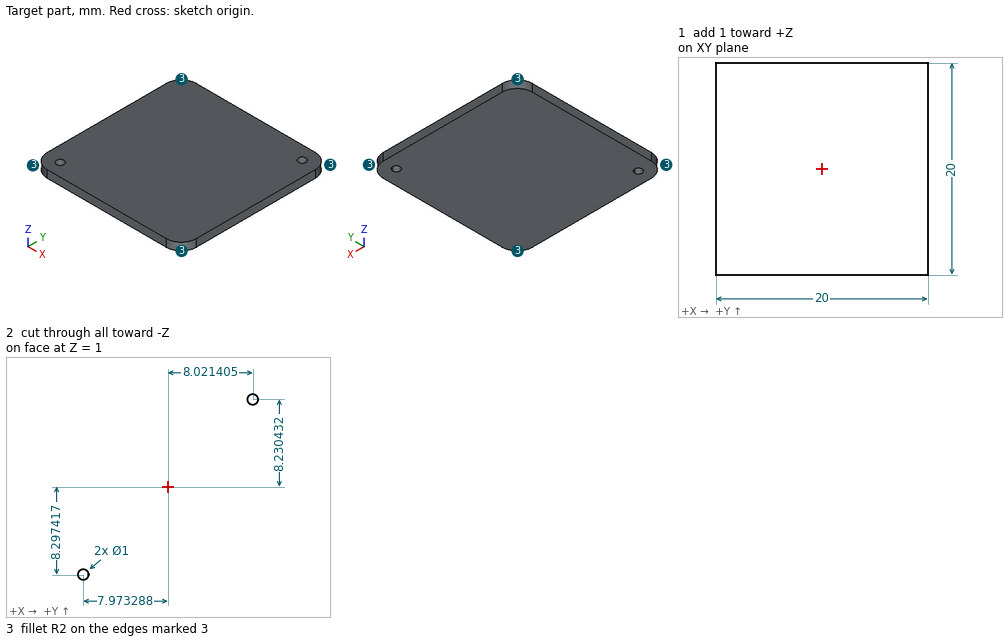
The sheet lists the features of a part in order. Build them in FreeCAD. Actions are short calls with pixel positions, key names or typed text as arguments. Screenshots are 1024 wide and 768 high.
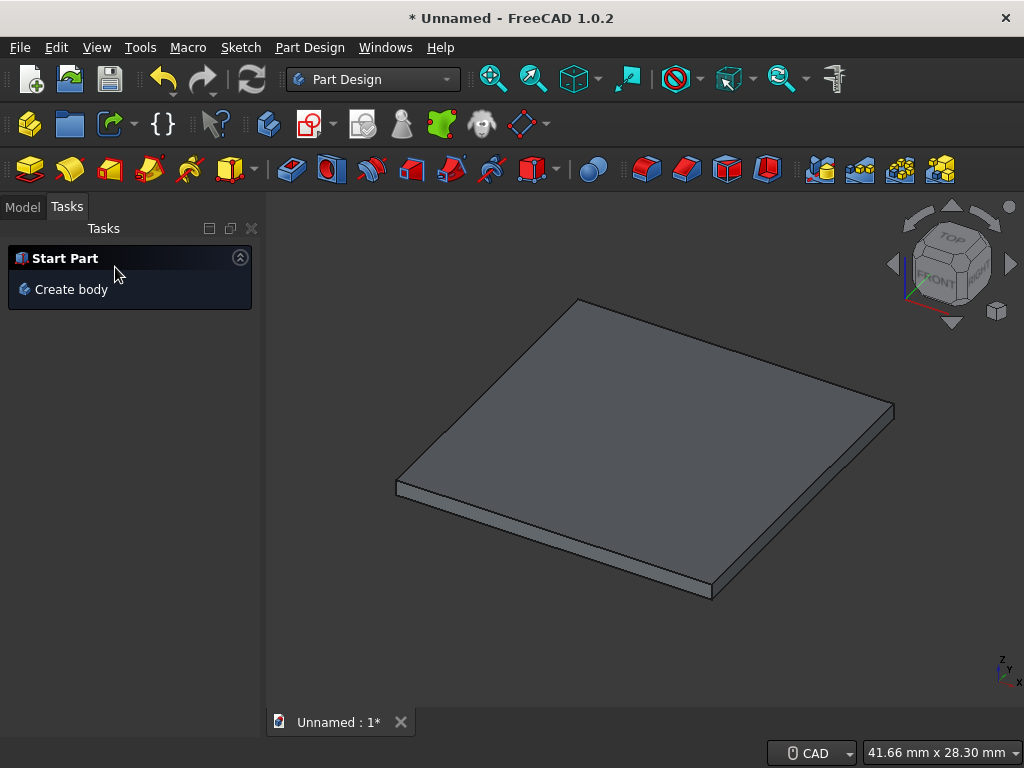
click(645, 441)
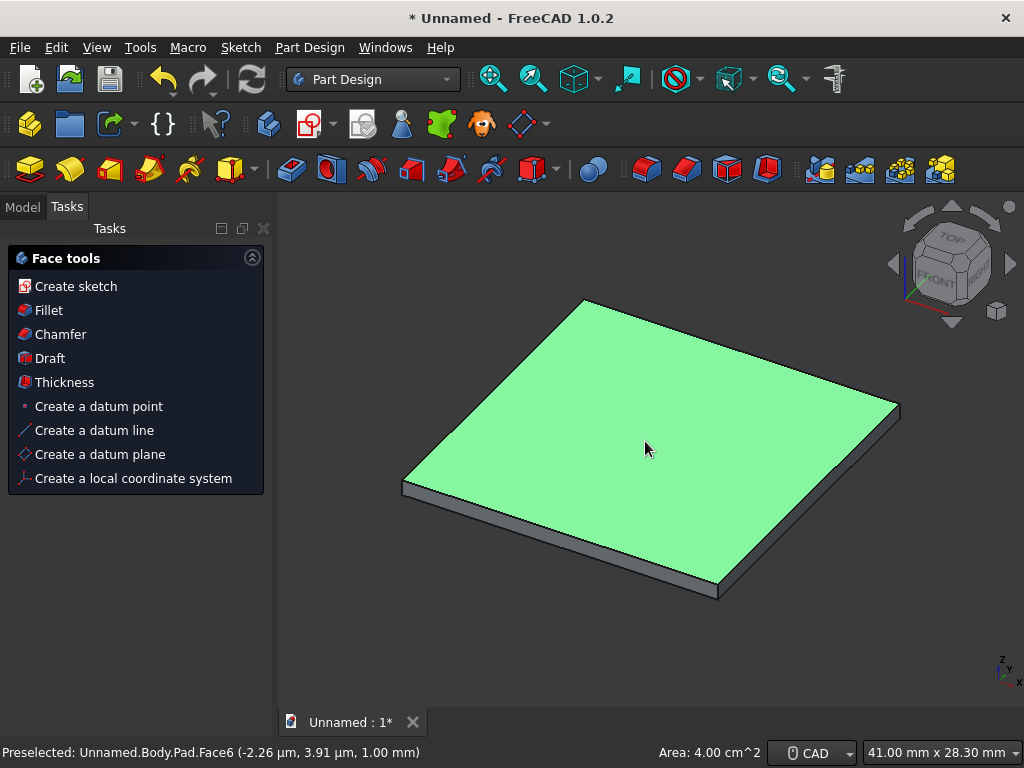
click(310, 124)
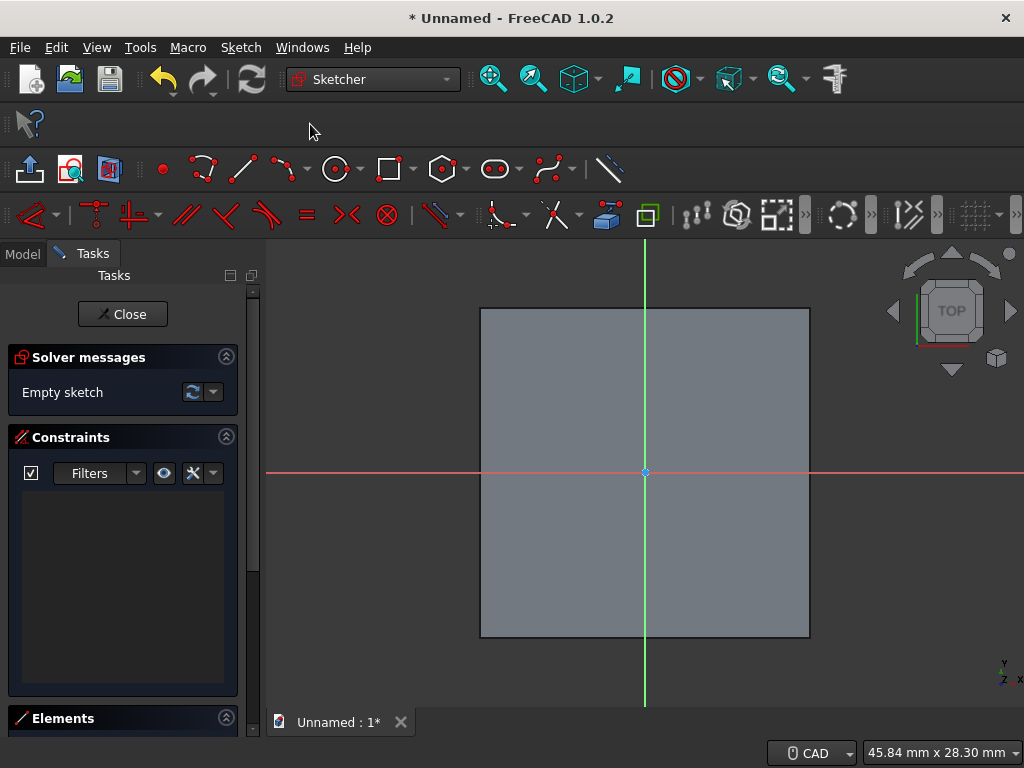
click(336, 170)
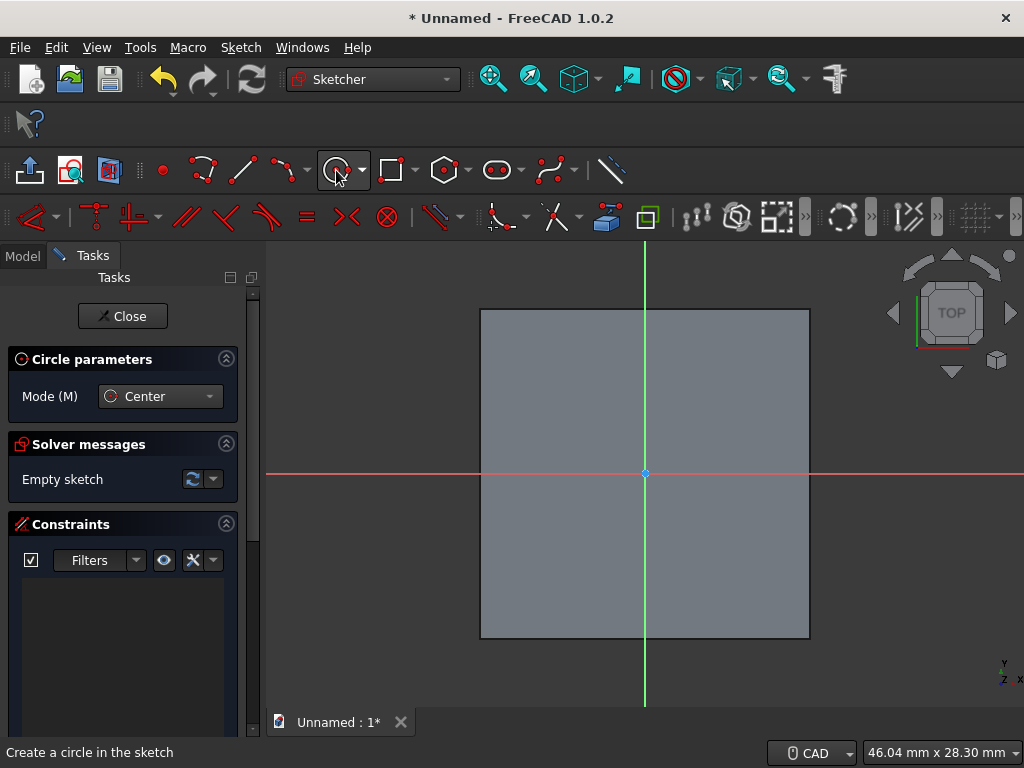
scroll(514, 611, up, 6)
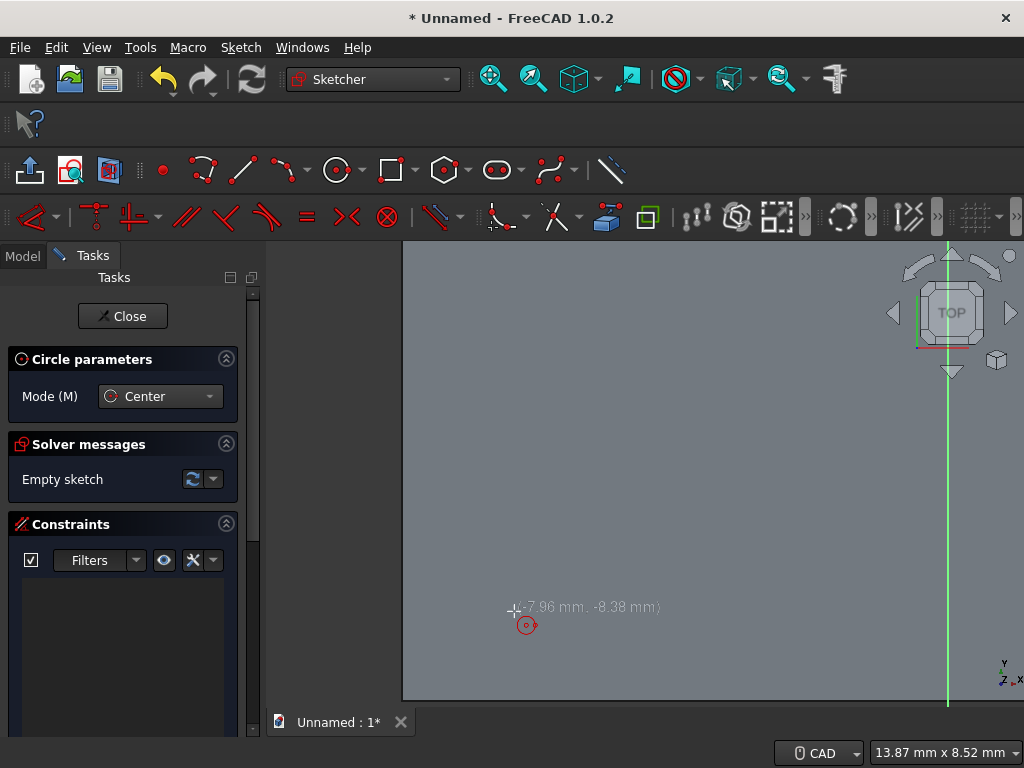
click(512, 608)
move(532, 589)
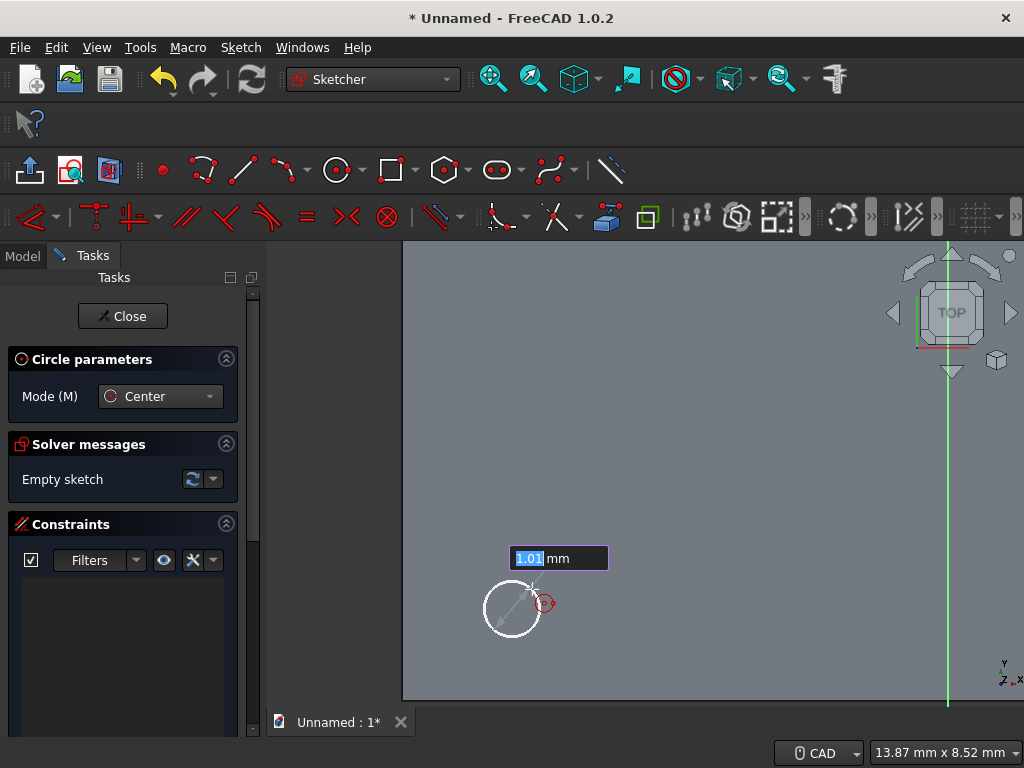
text(1)
key(Return)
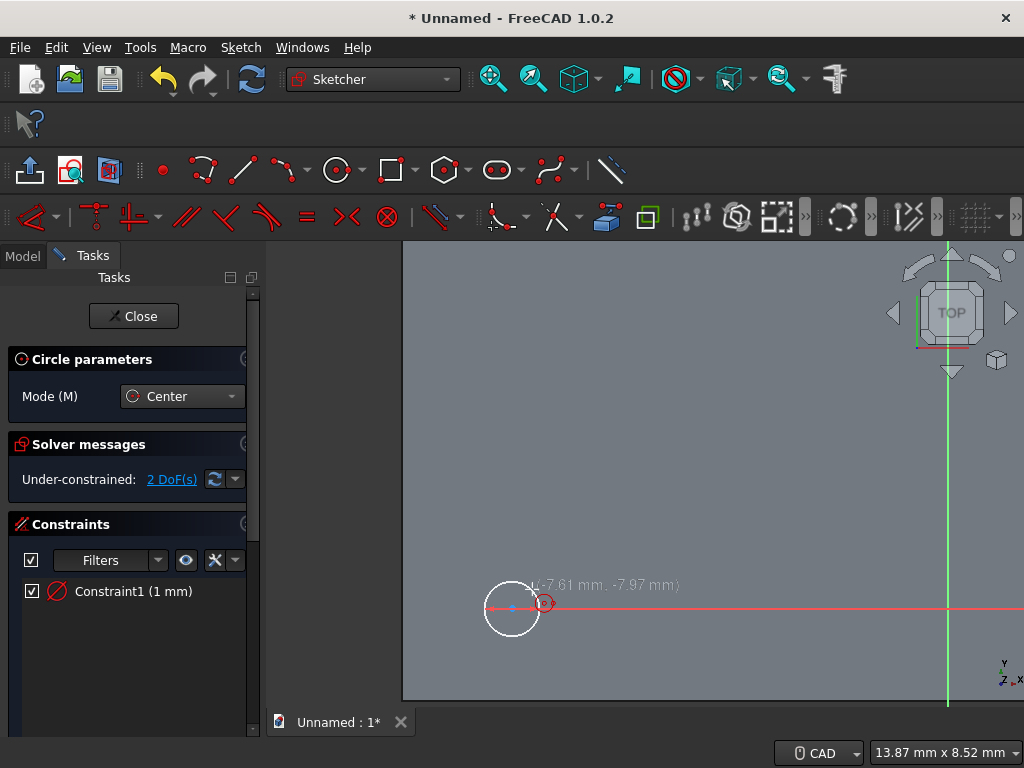
scroll(416, 611, down, 6)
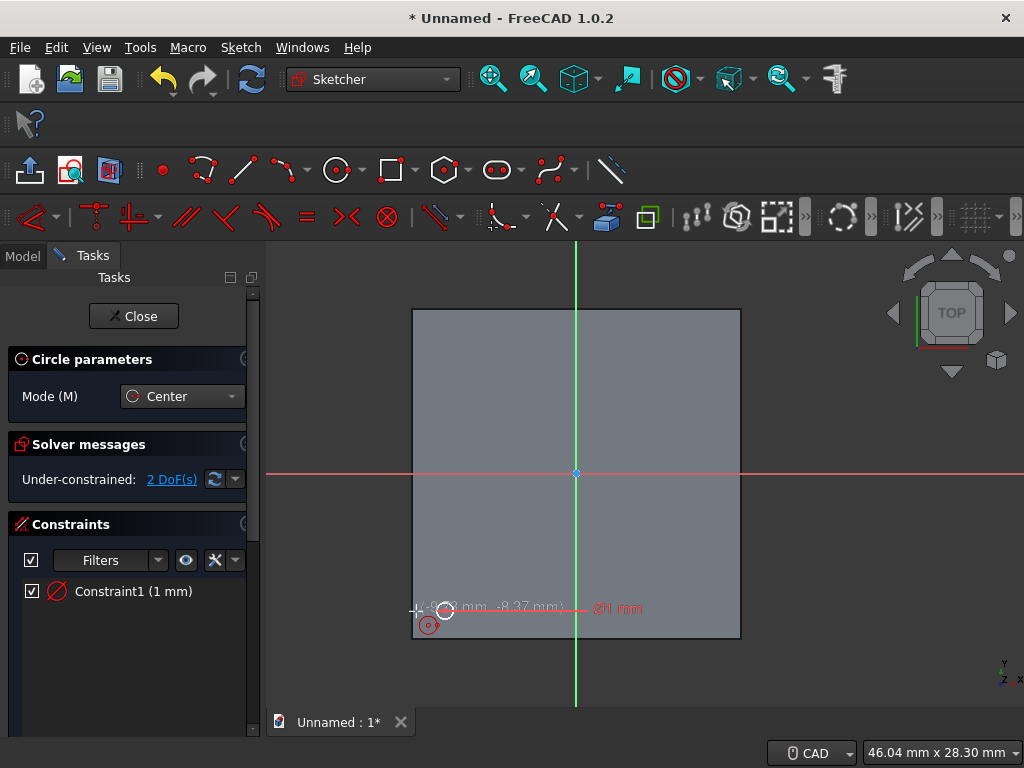
scroll(709, 338, up, 6)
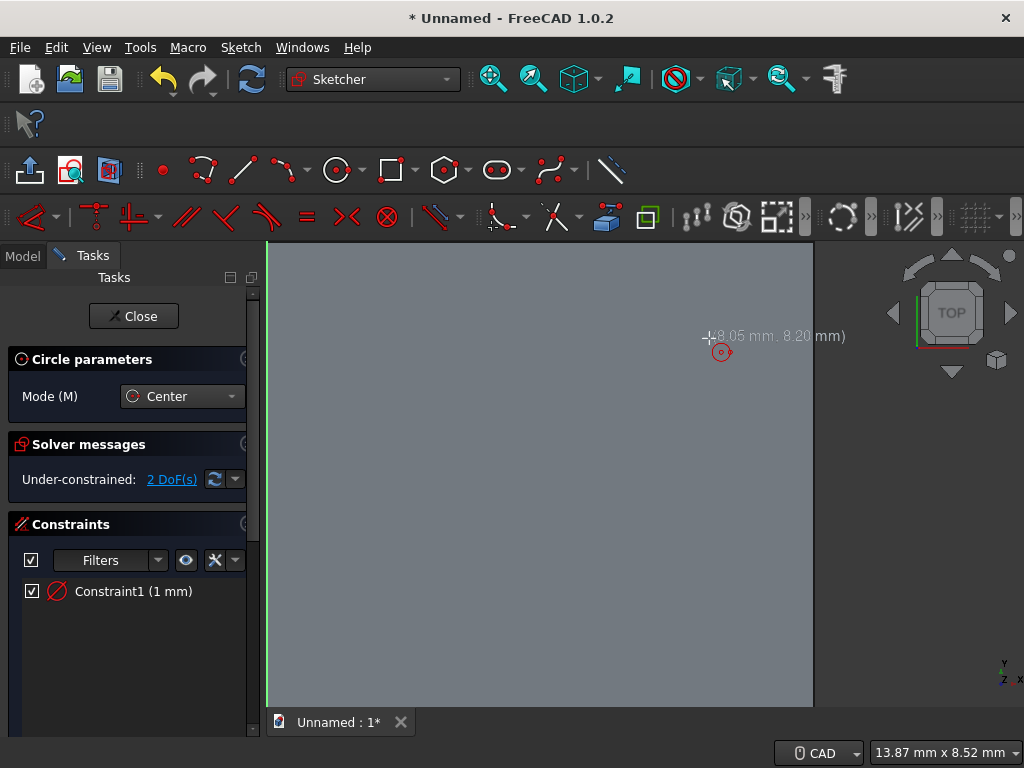
click(706, 339)
move(725, 320)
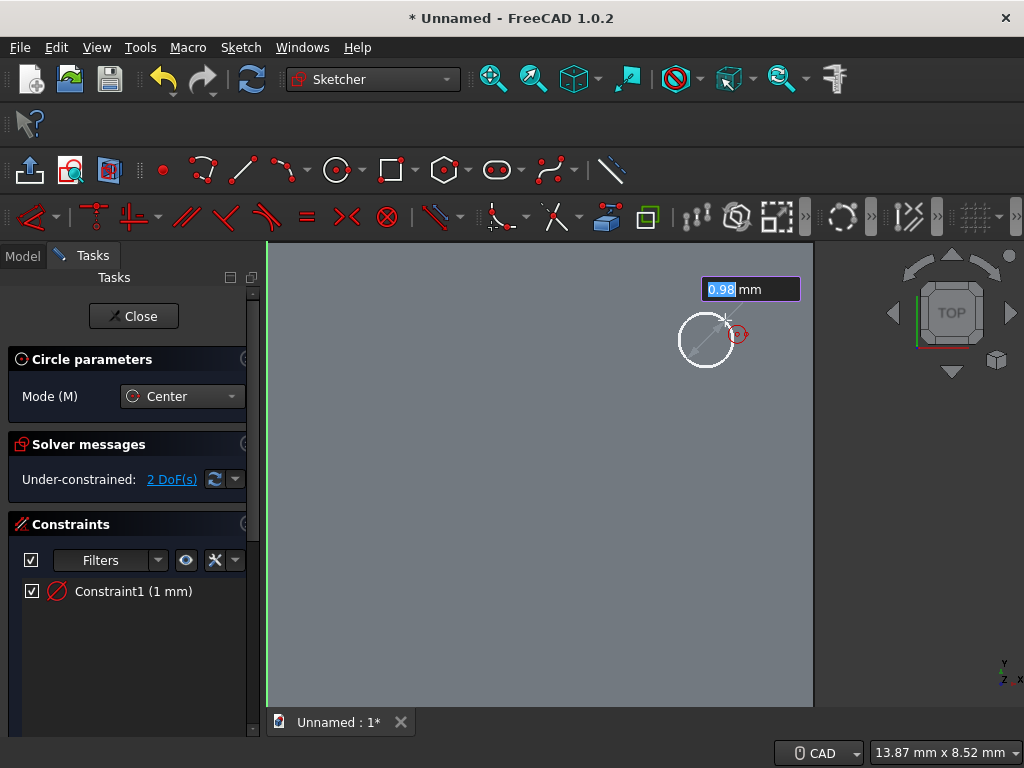
text(1)
key(Return)
key(Escape)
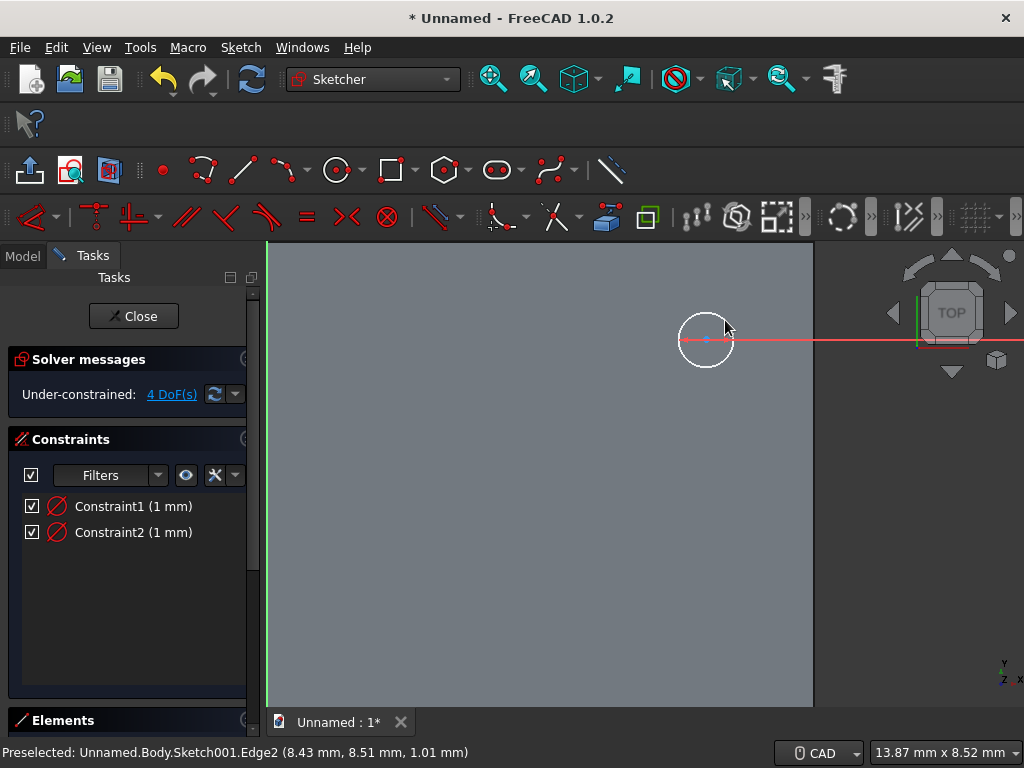
key(d)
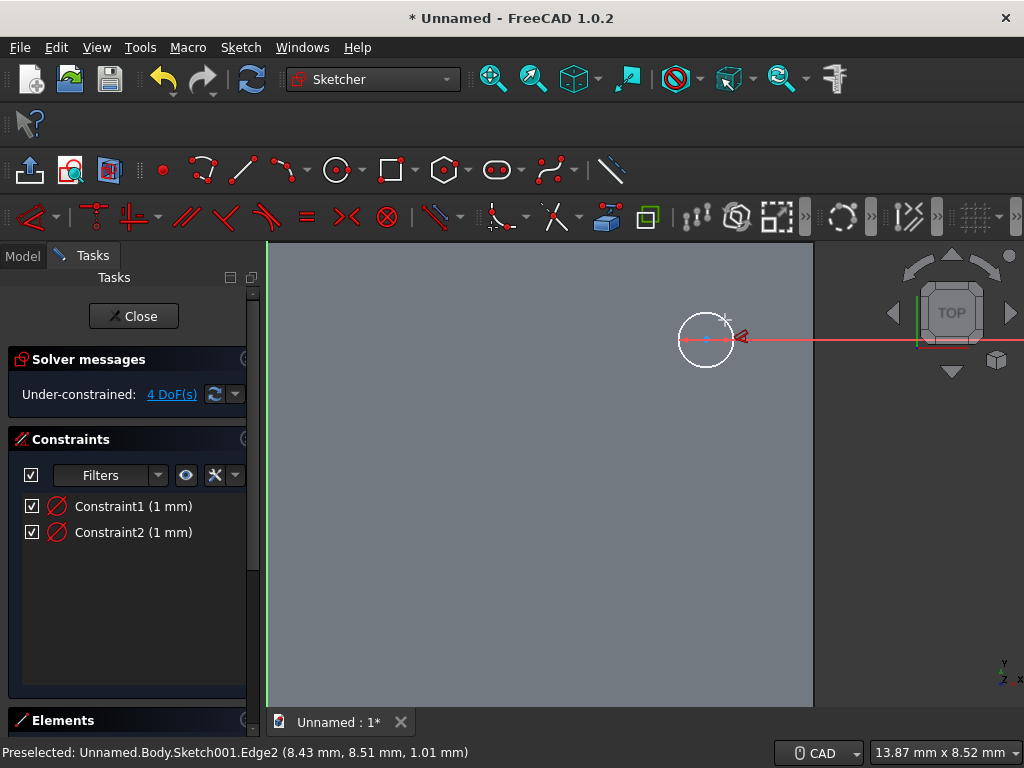
scroll(709, 337, down, 6)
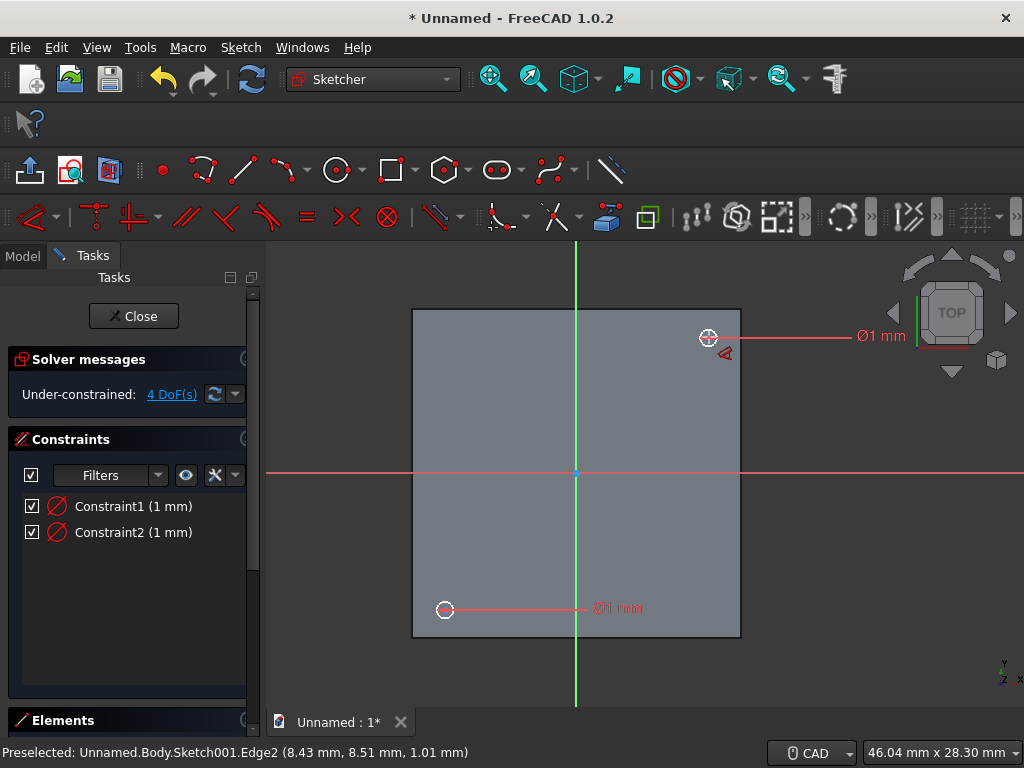
click(445, 610)
click(511, 644)